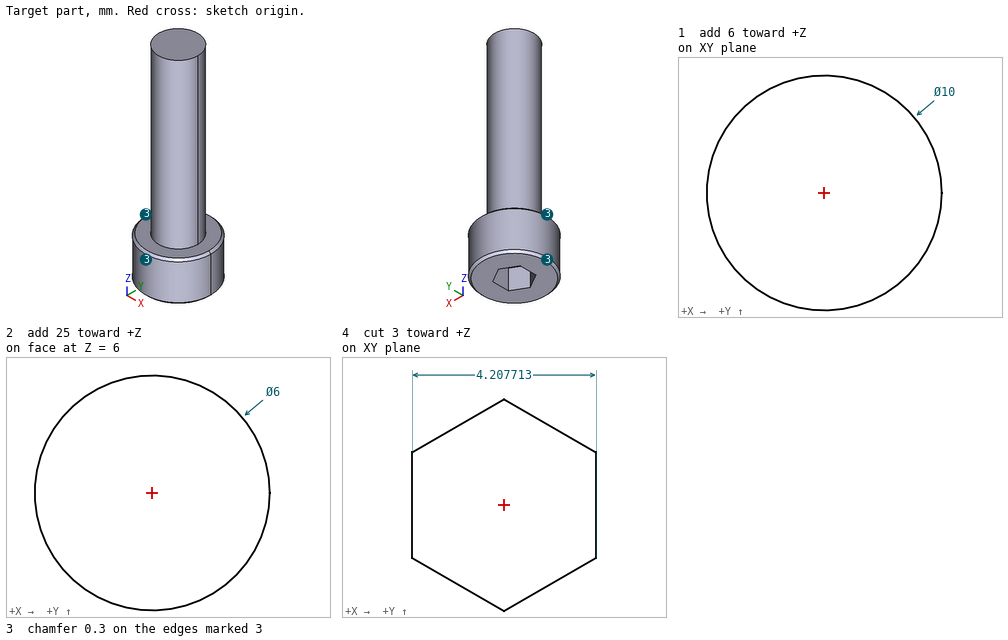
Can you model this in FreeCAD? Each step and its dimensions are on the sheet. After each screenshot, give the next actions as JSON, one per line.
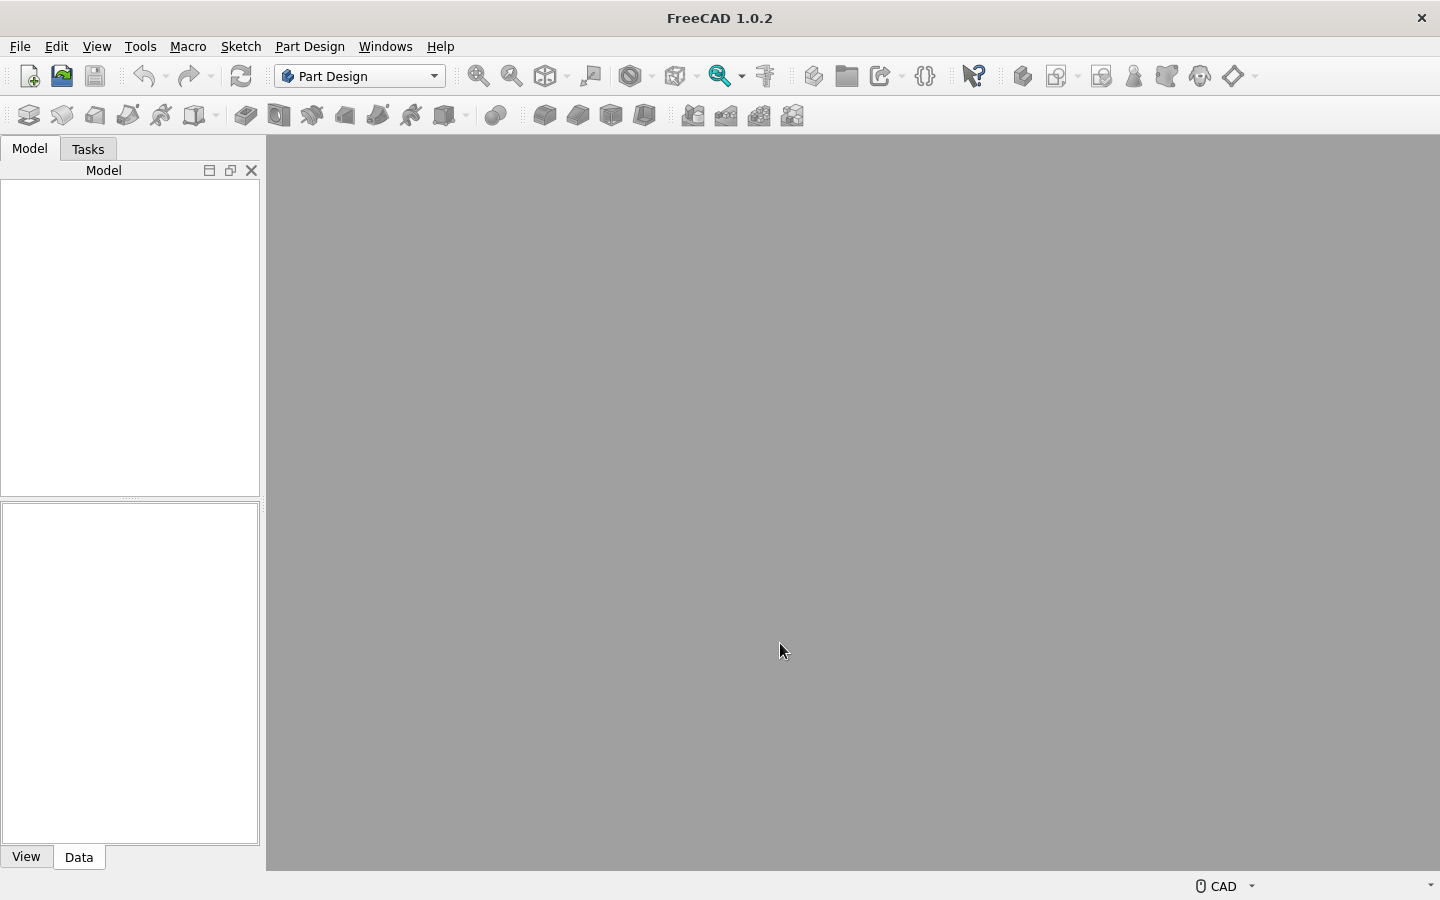
{"action": "left_click", "coordinate": [29, 76]}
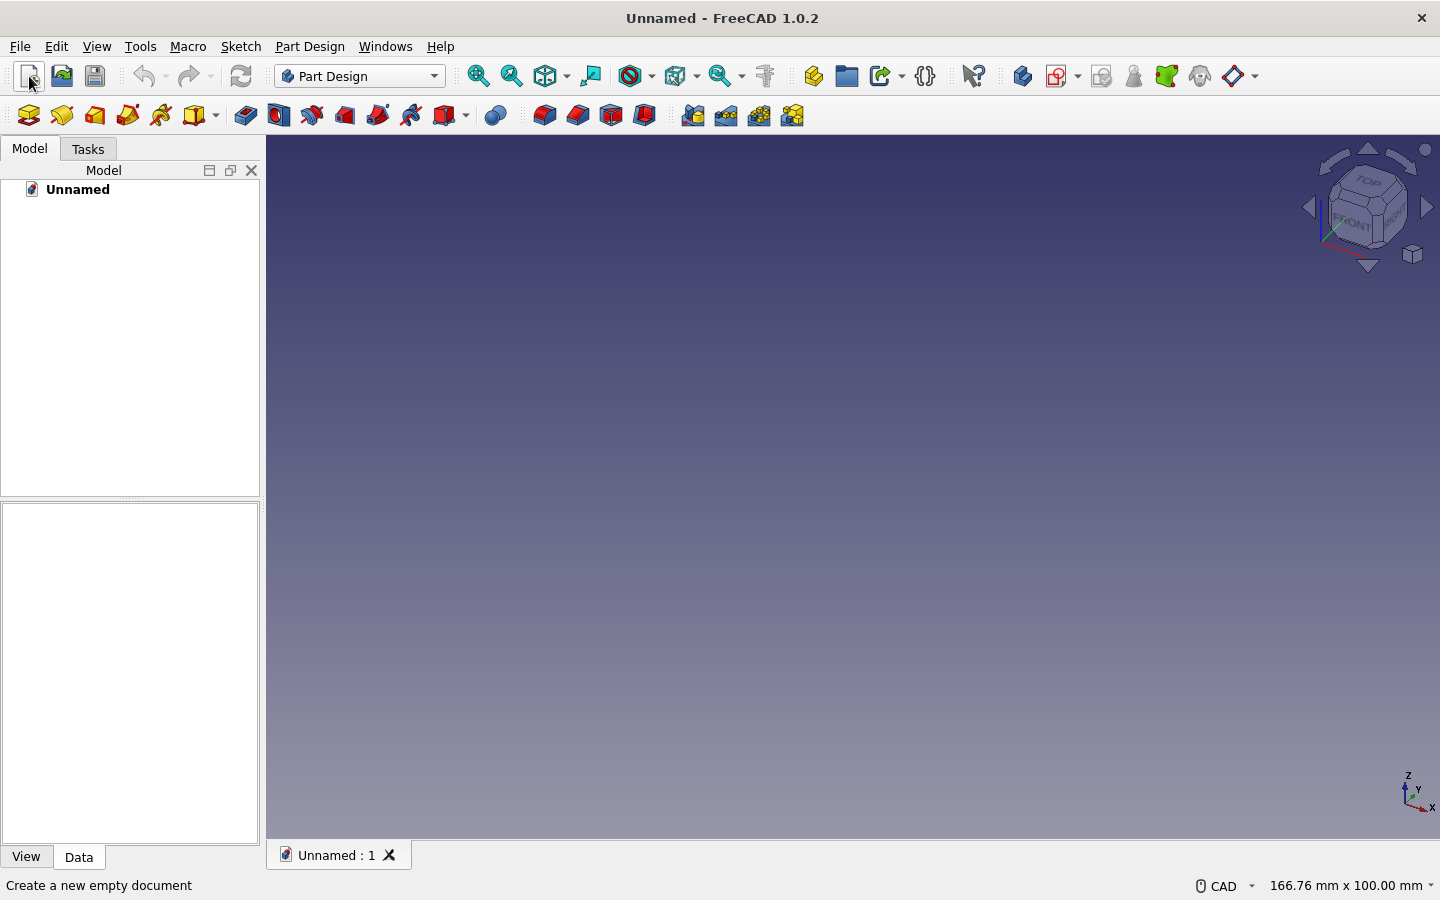
{"action": "left_click", "coordinate": [1056, 76]}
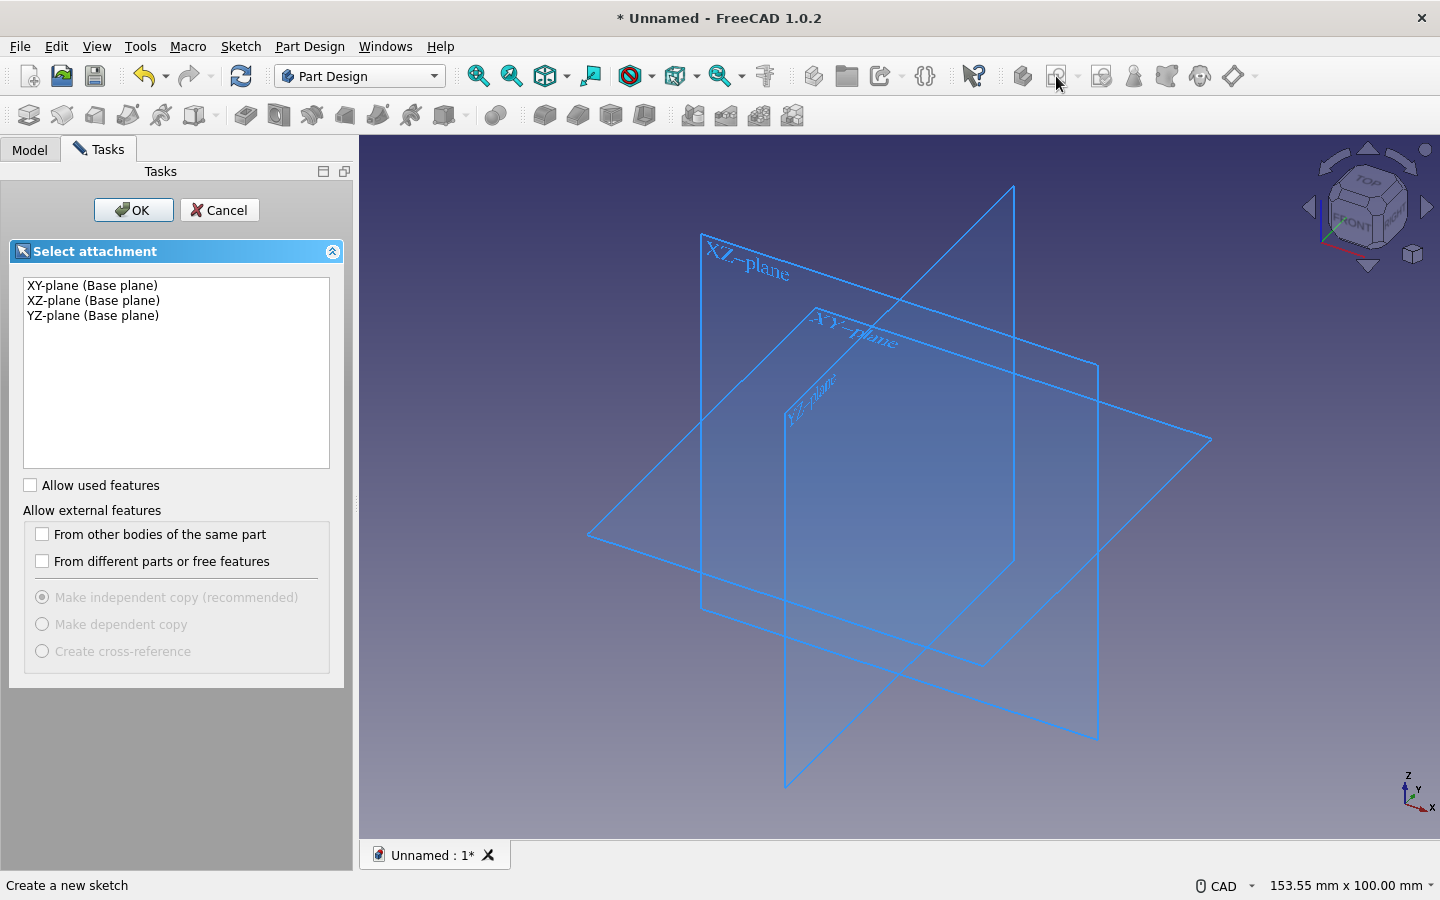
{"action": "left_click", "coordinate": [84, 286]}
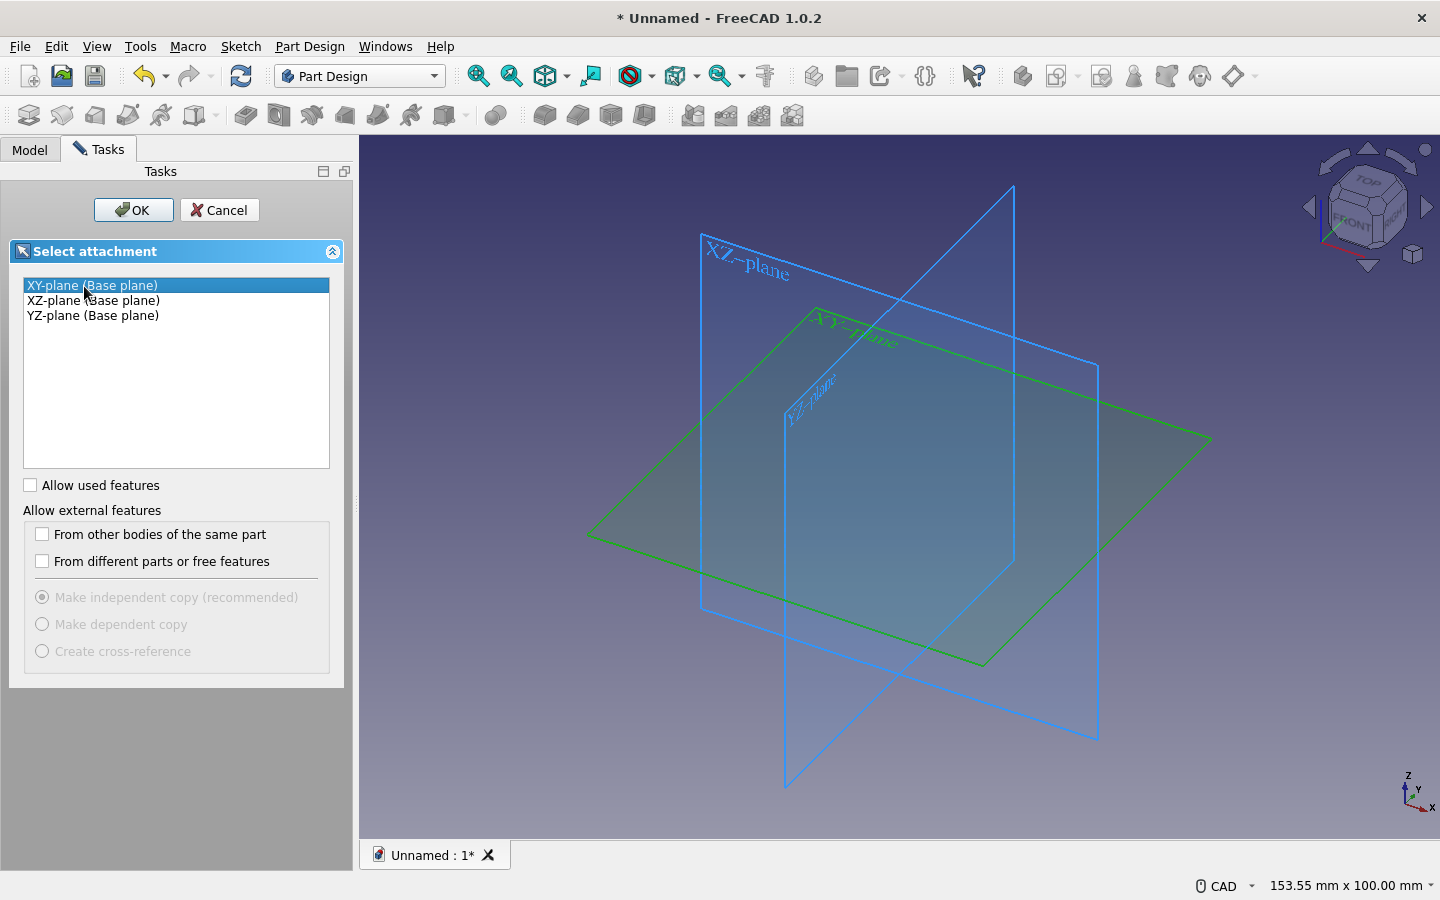
{"action": "left_click", "coordinate": [134, 210]}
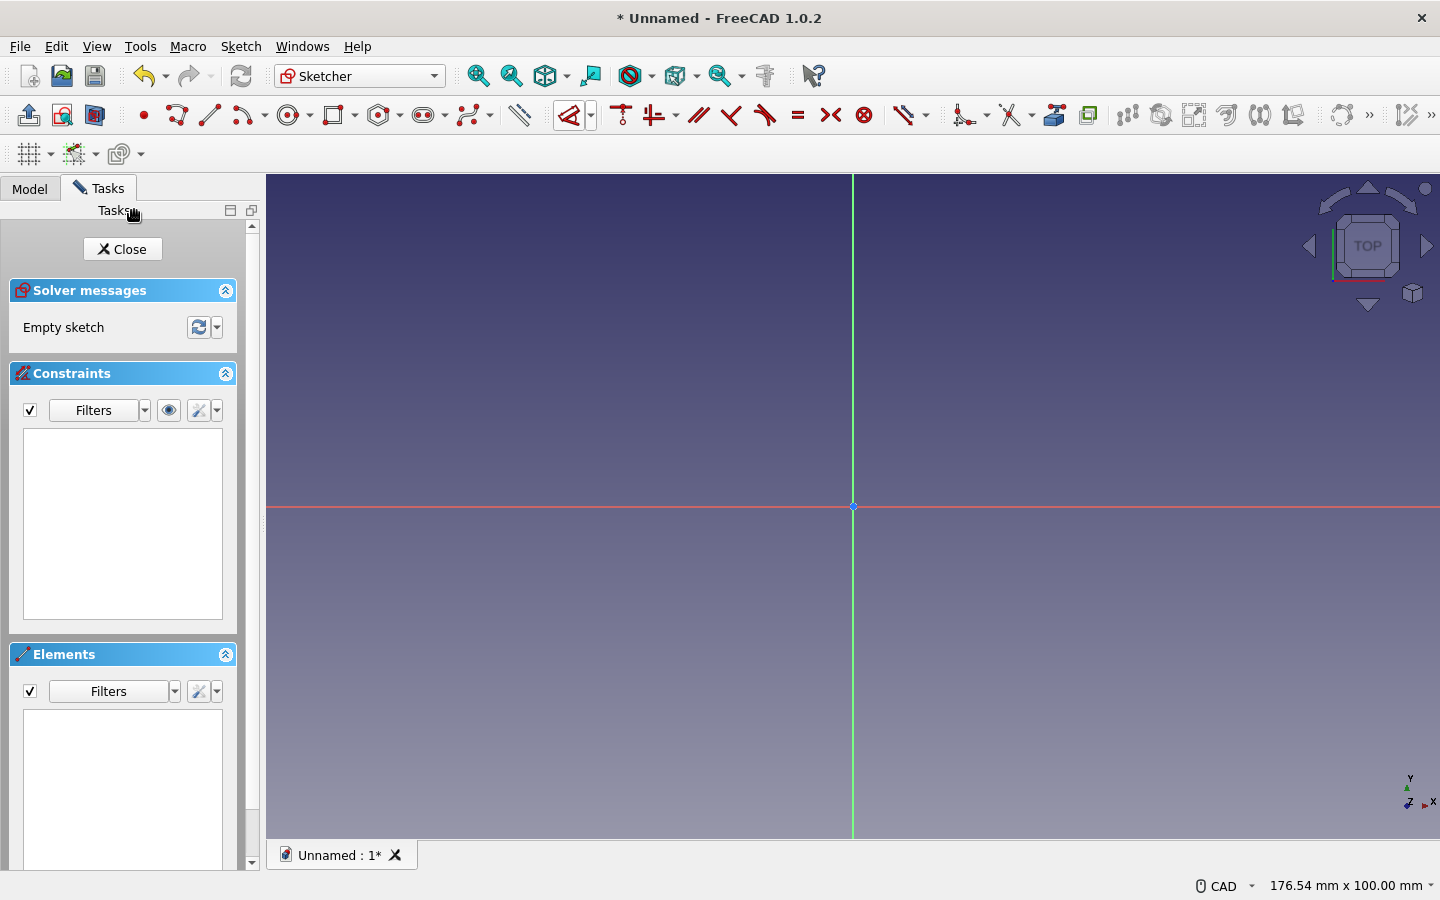
{"action": "scroll", "coordinate": [867, 506], "scroll_direction": "up", "scroll_amount": 9}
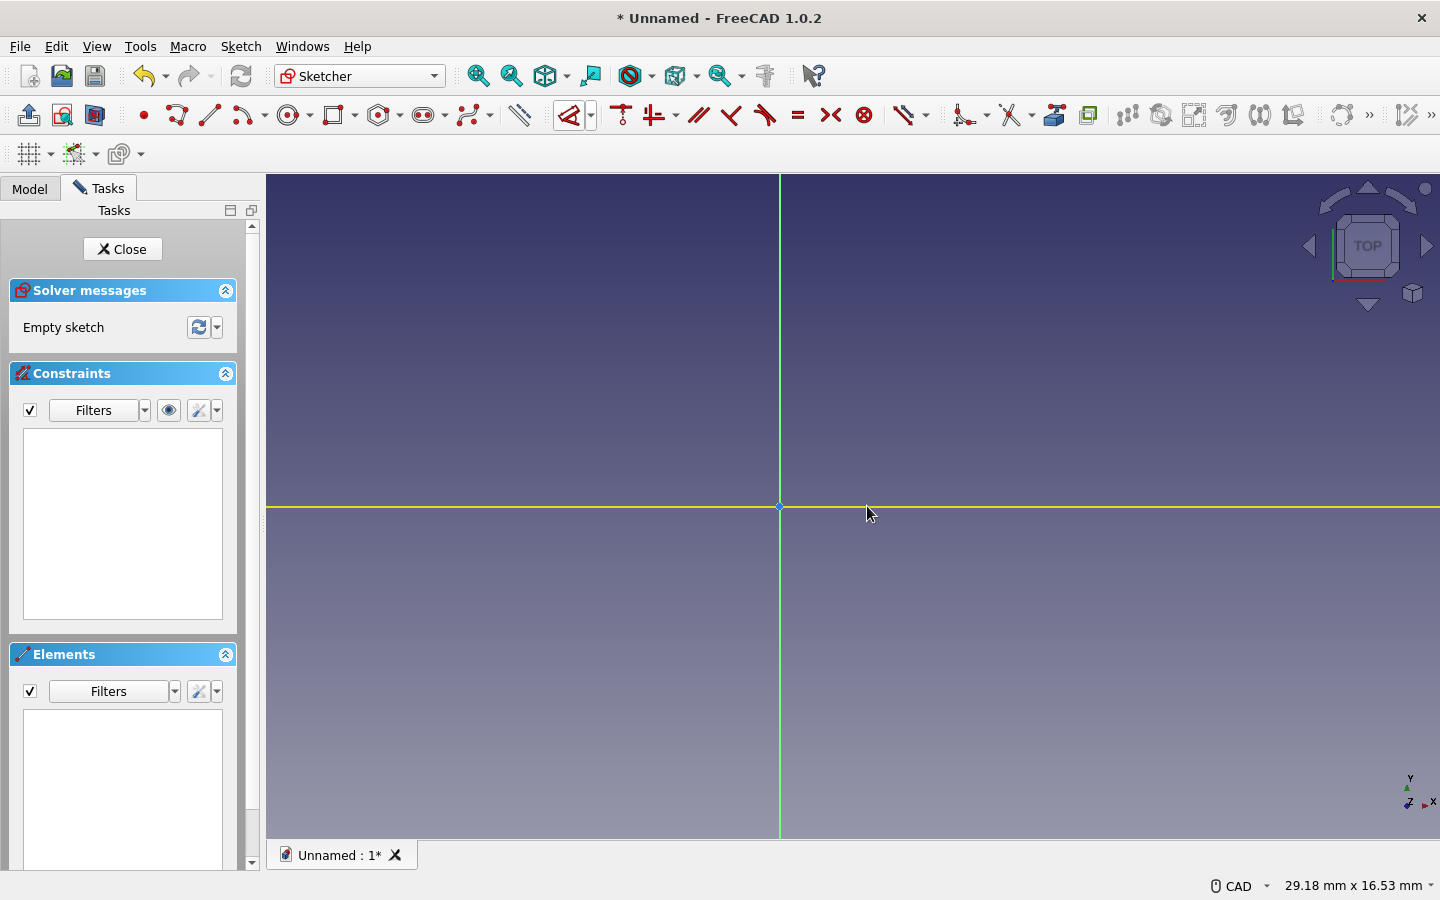
{"action": "key", "text": "g c"}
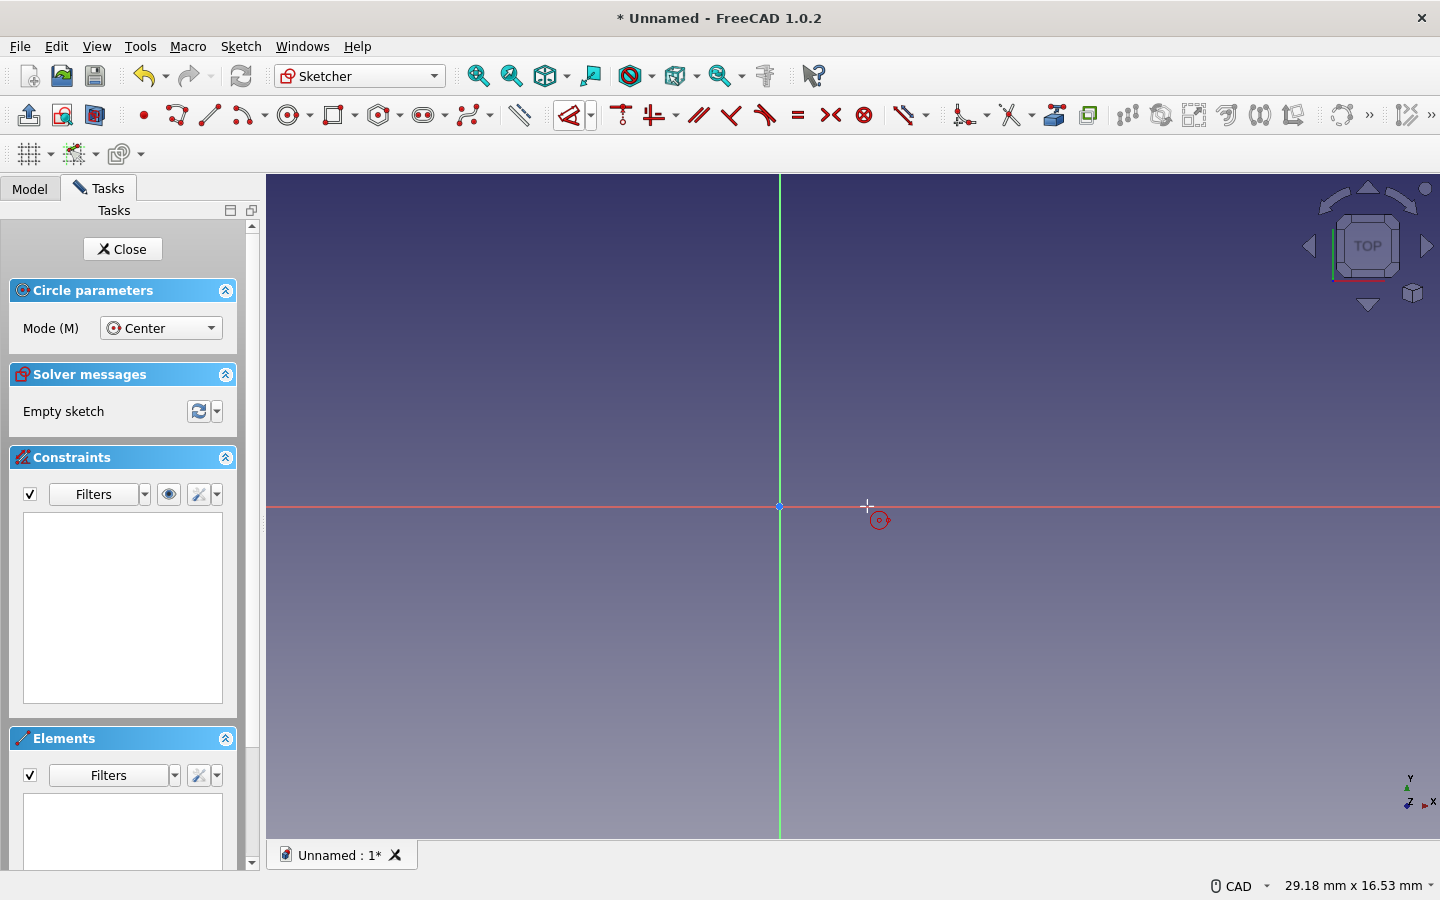
{"action": "left_click", "coordinate": [780, 506]}
{"action": "mouse_move", "coordinate": [922, 364]}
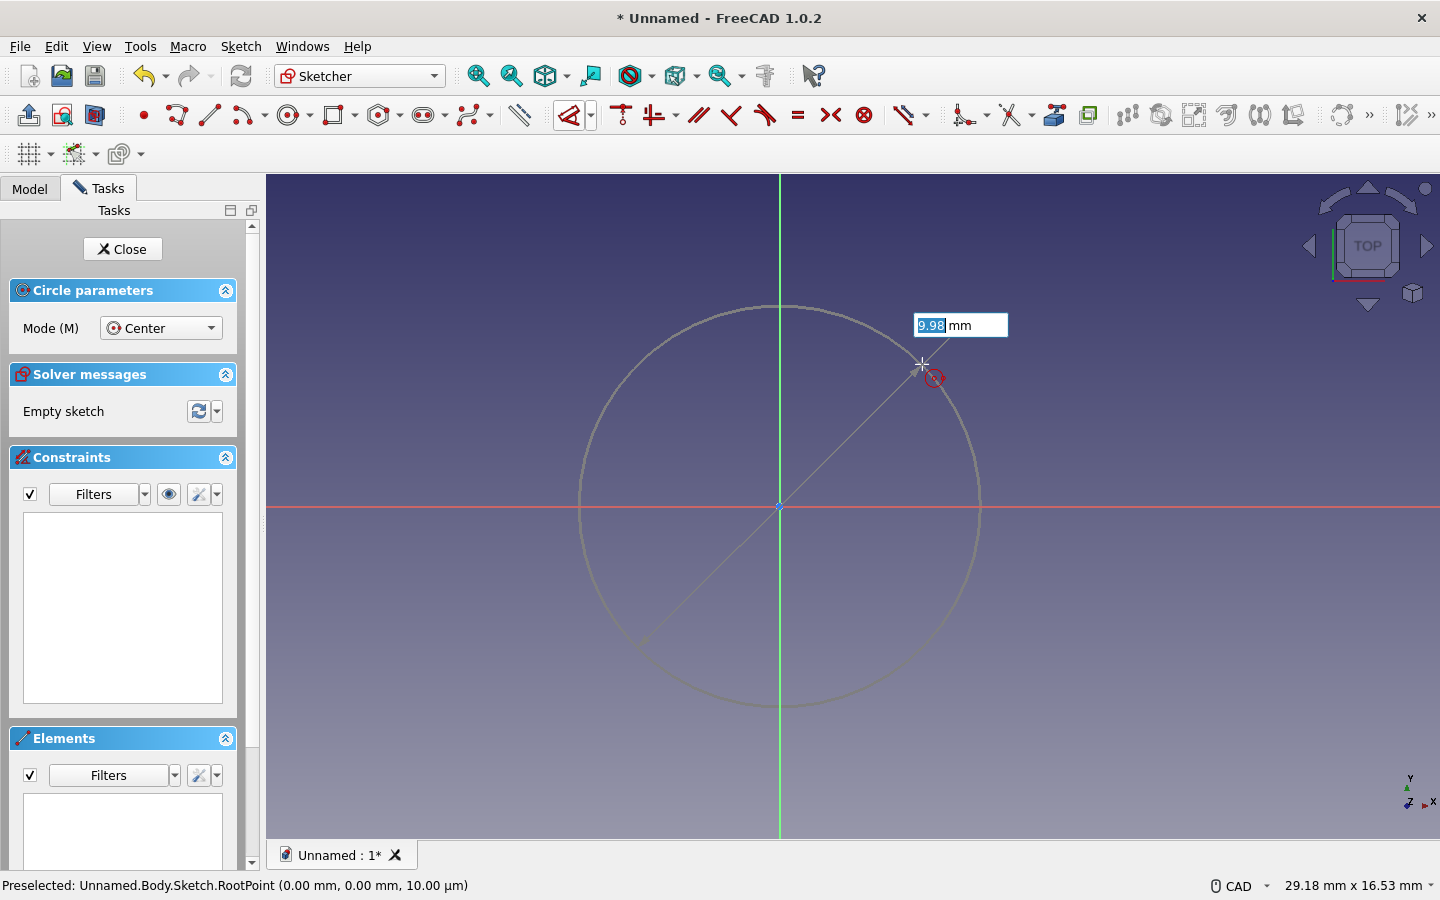
{"action": "type", "text": "10"}
{"action": "key", "text": "Return"}
{"action": "key", "text": "Escape"}